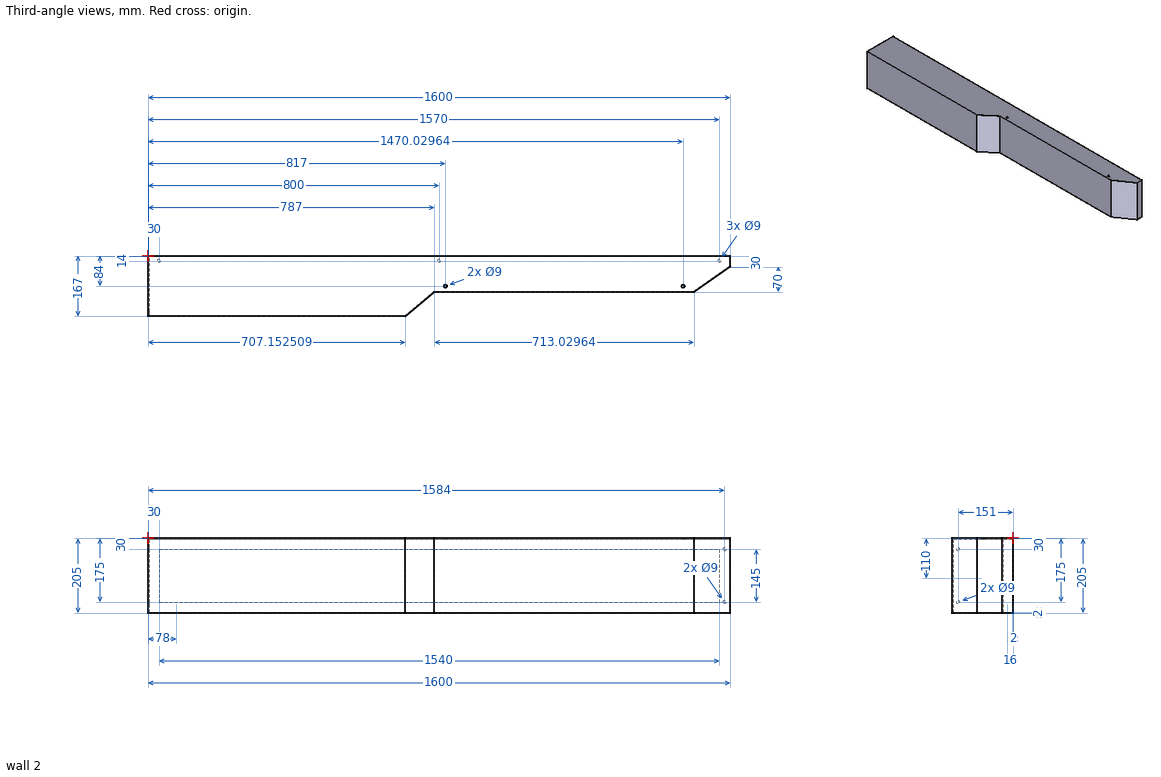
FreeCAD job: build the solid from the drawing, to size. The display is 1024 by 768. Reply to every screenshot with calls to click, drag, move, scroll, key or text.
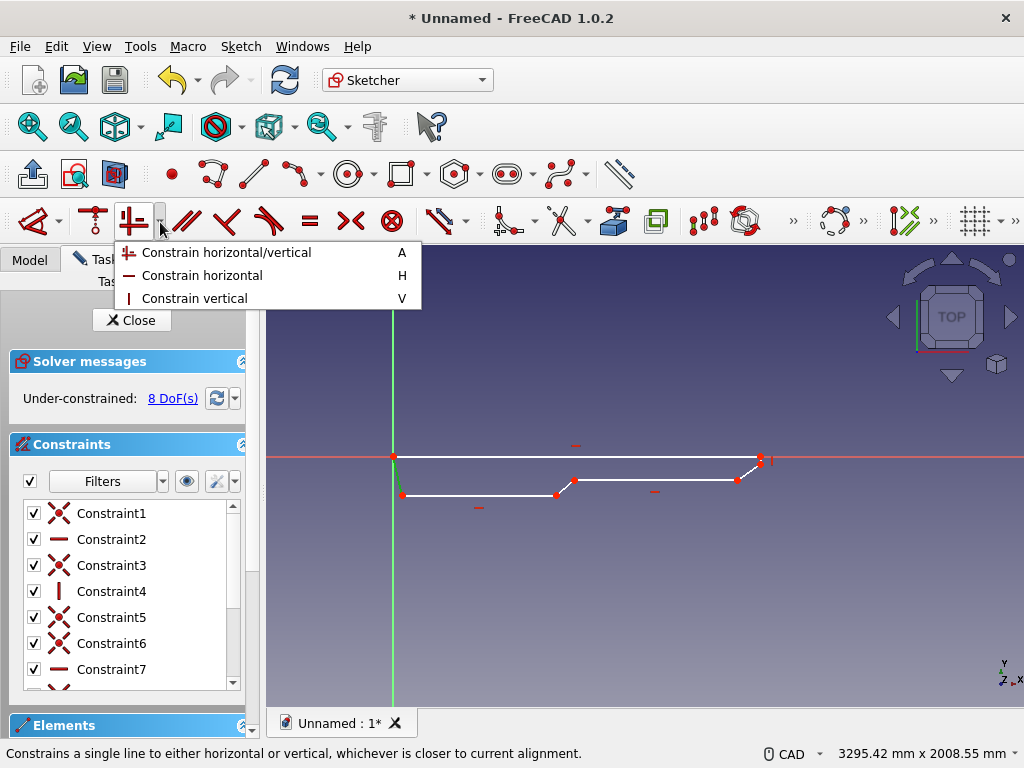
click(268, 298)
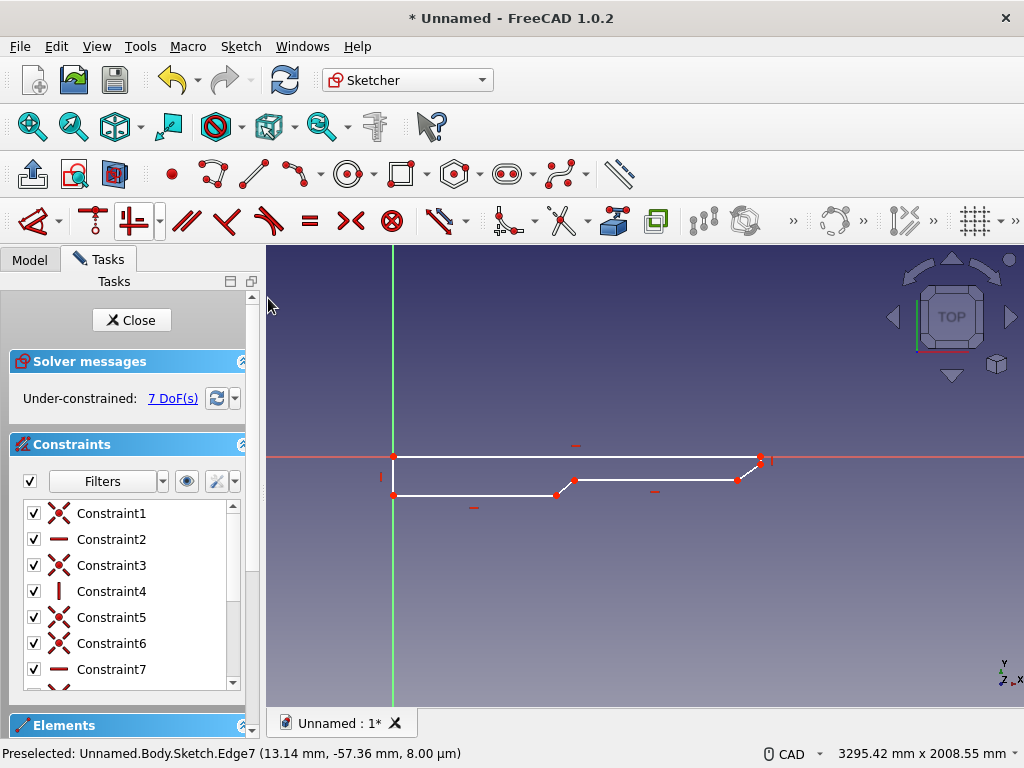
key(d)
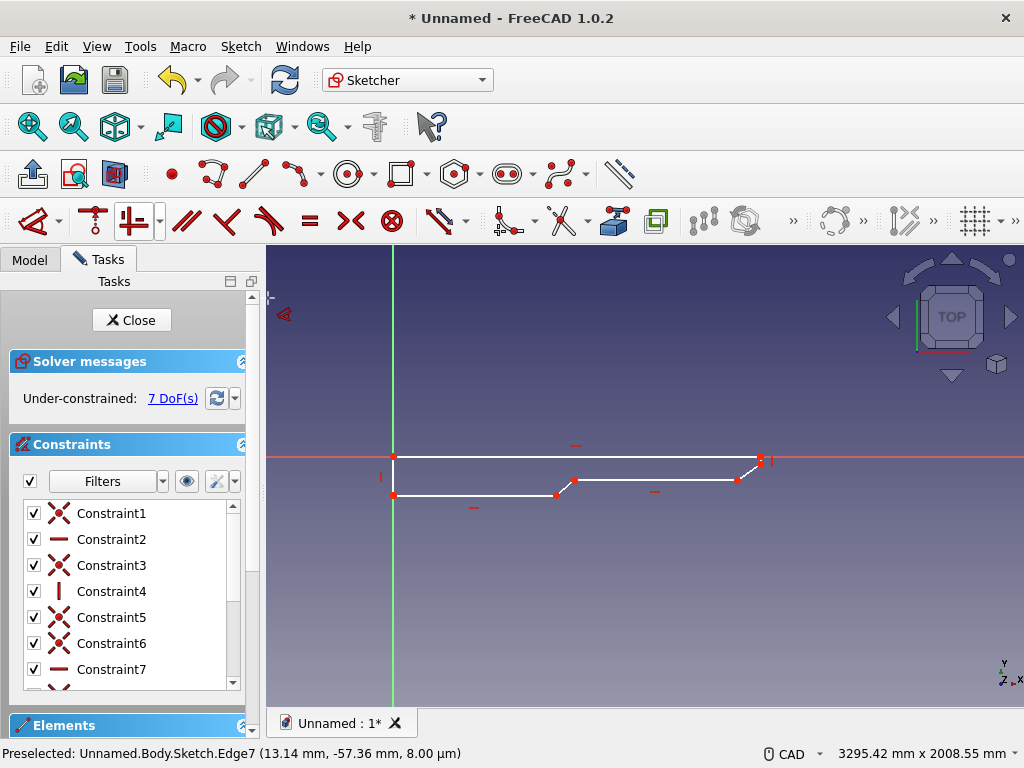
scroll(761, 460, up, 9)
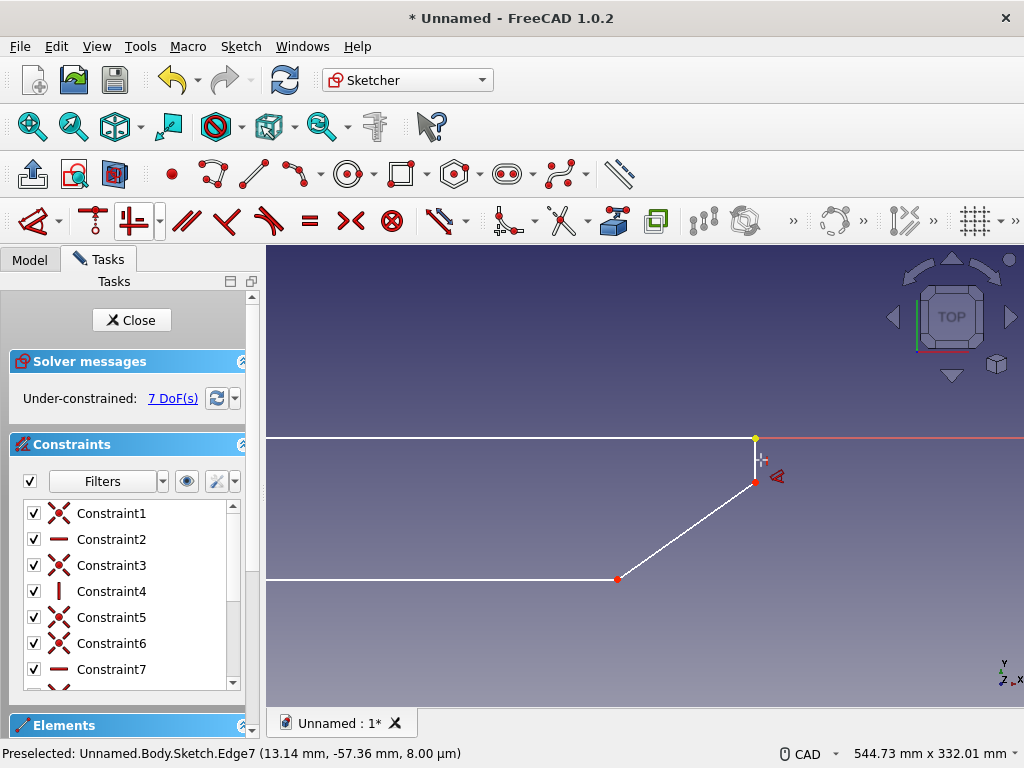
click(755, 460)
click(789, 460)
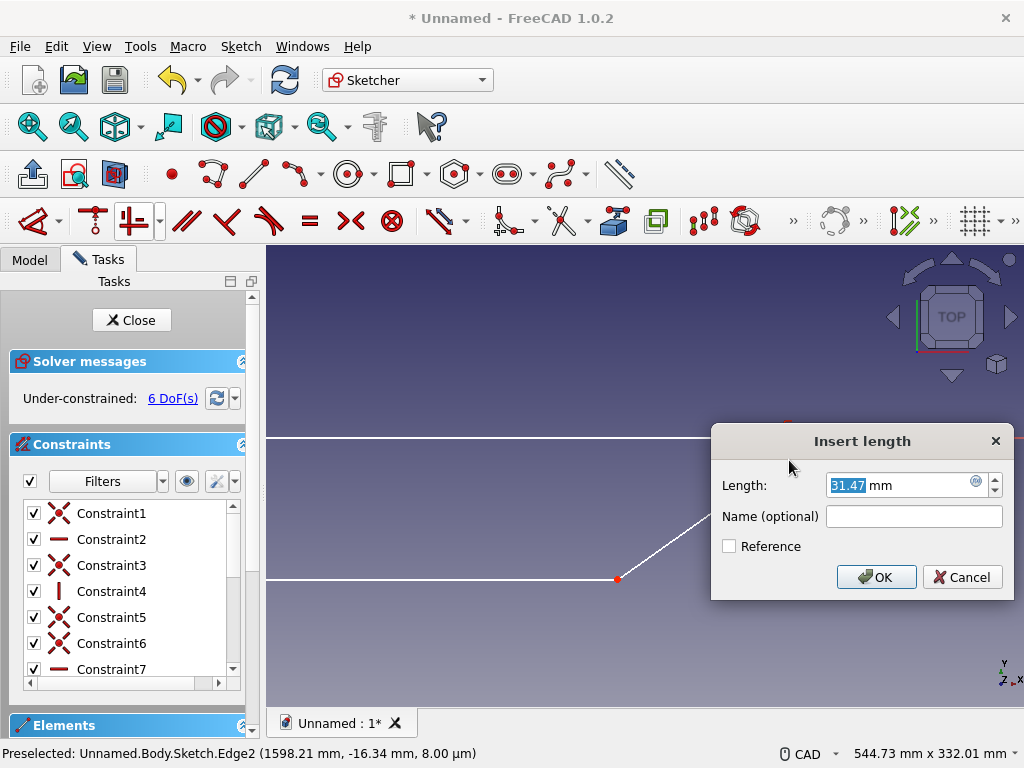
text(30)
key(Return)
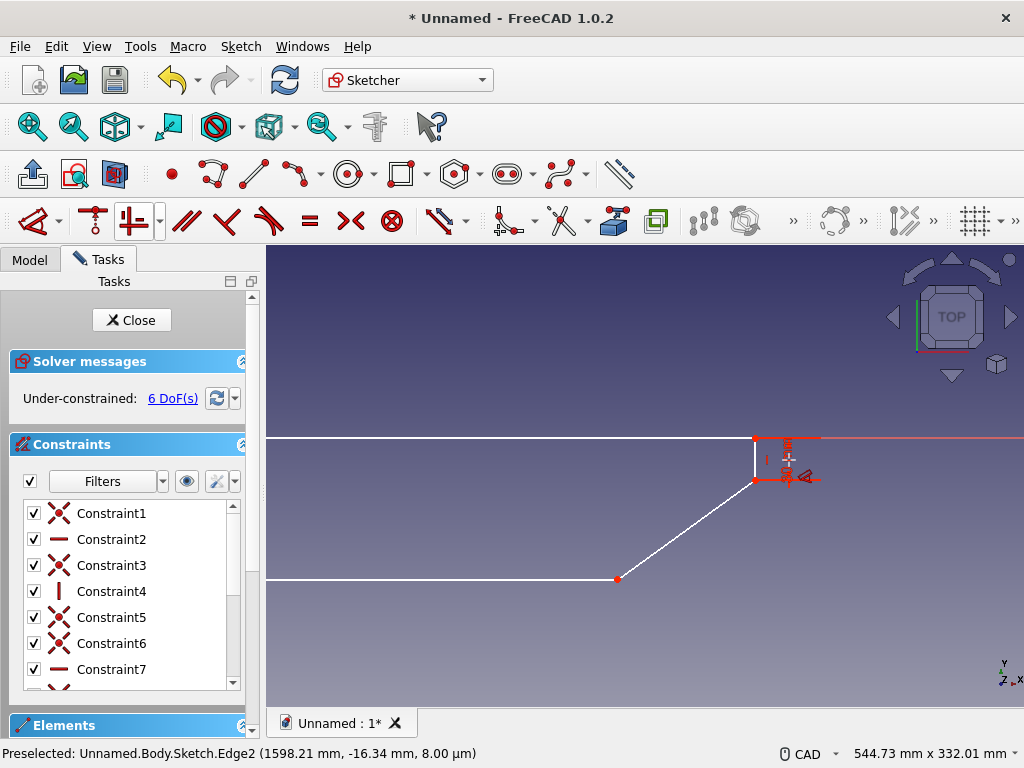
scroll(761, 460, down, 9)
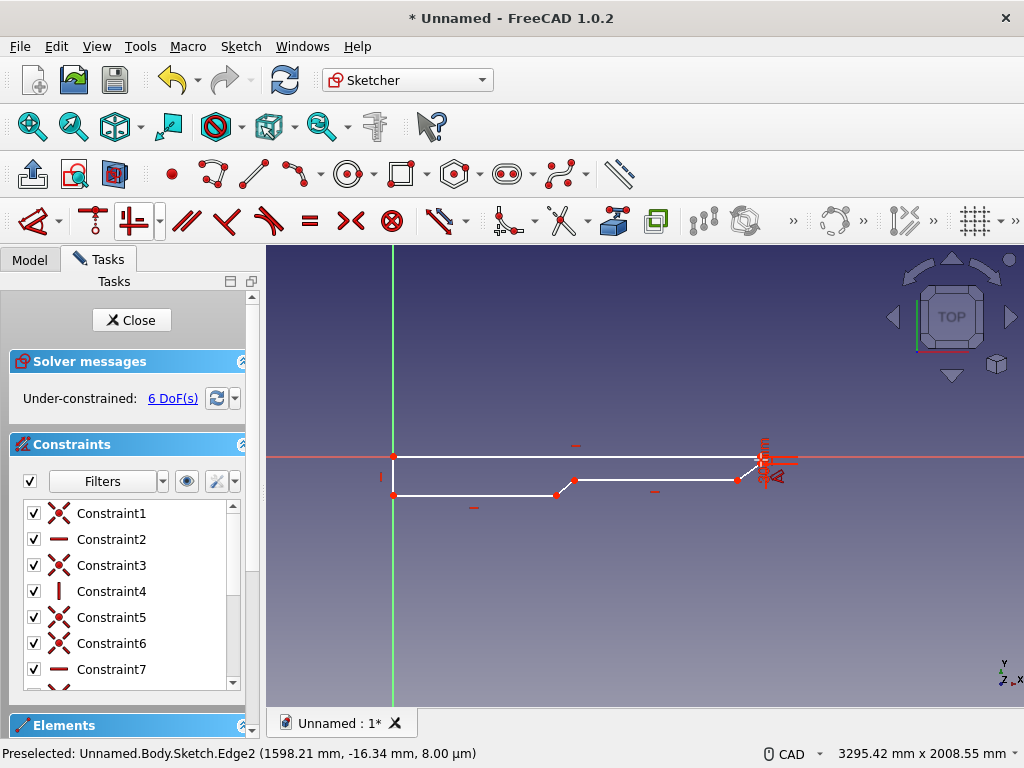
click(393, 484)
click(359, 476)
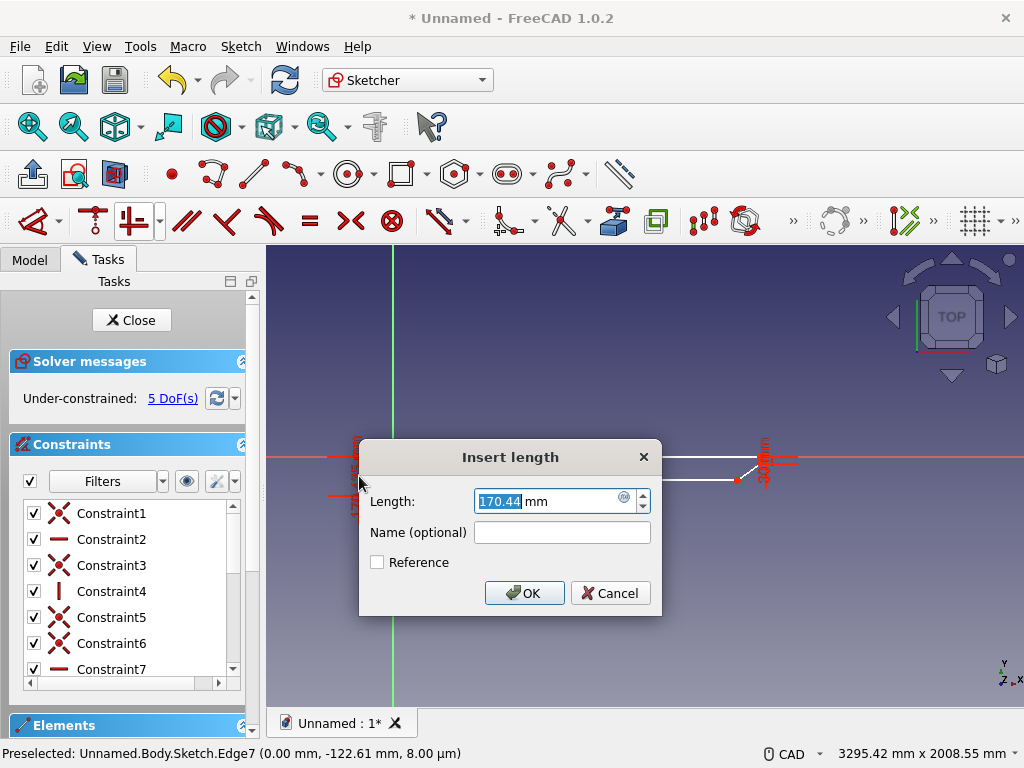
text(167)
key(Return)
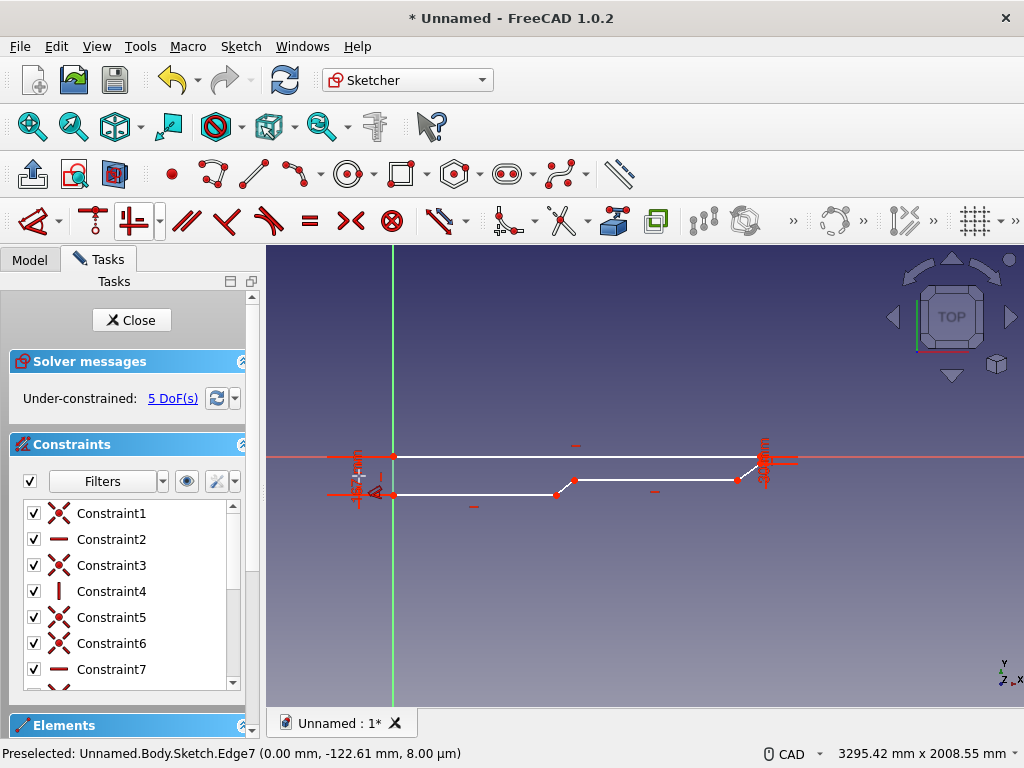
scroll(752, 470, up, 5)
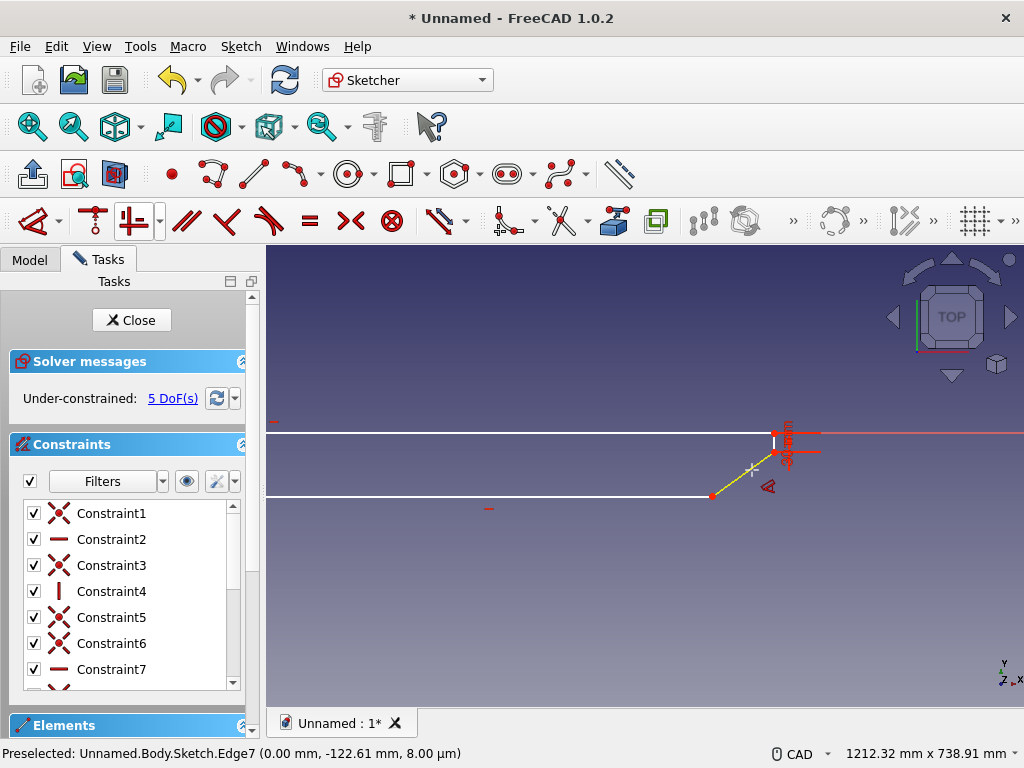
click(750, 470)
click(808, 474)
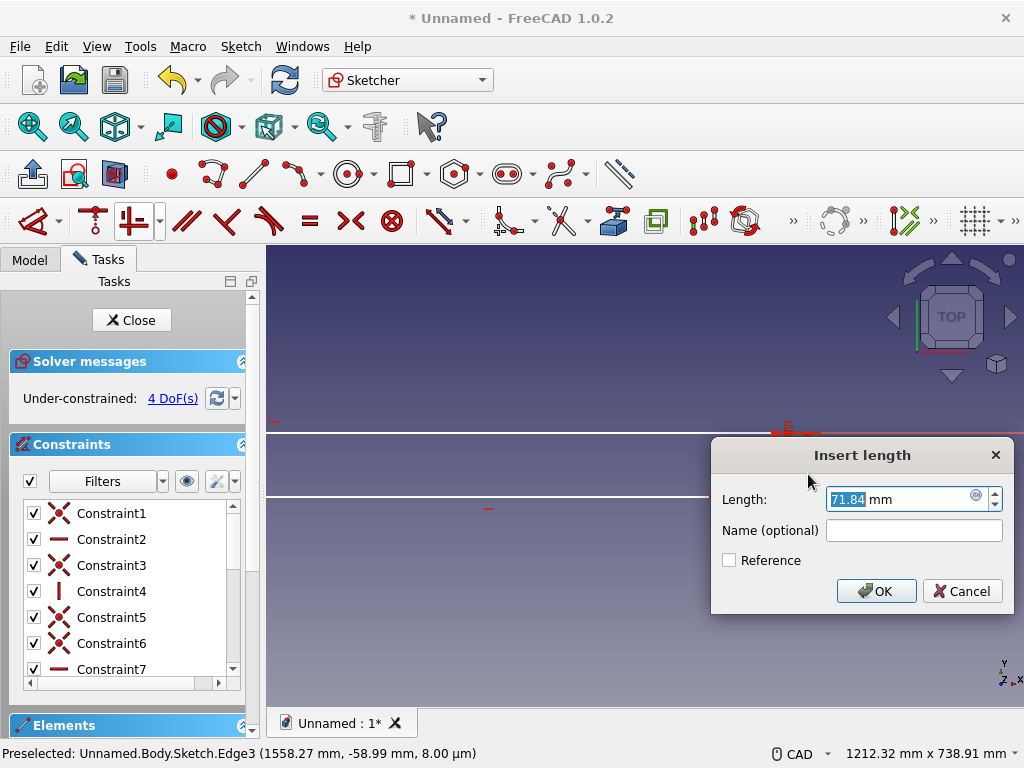
text(70)
key(Return)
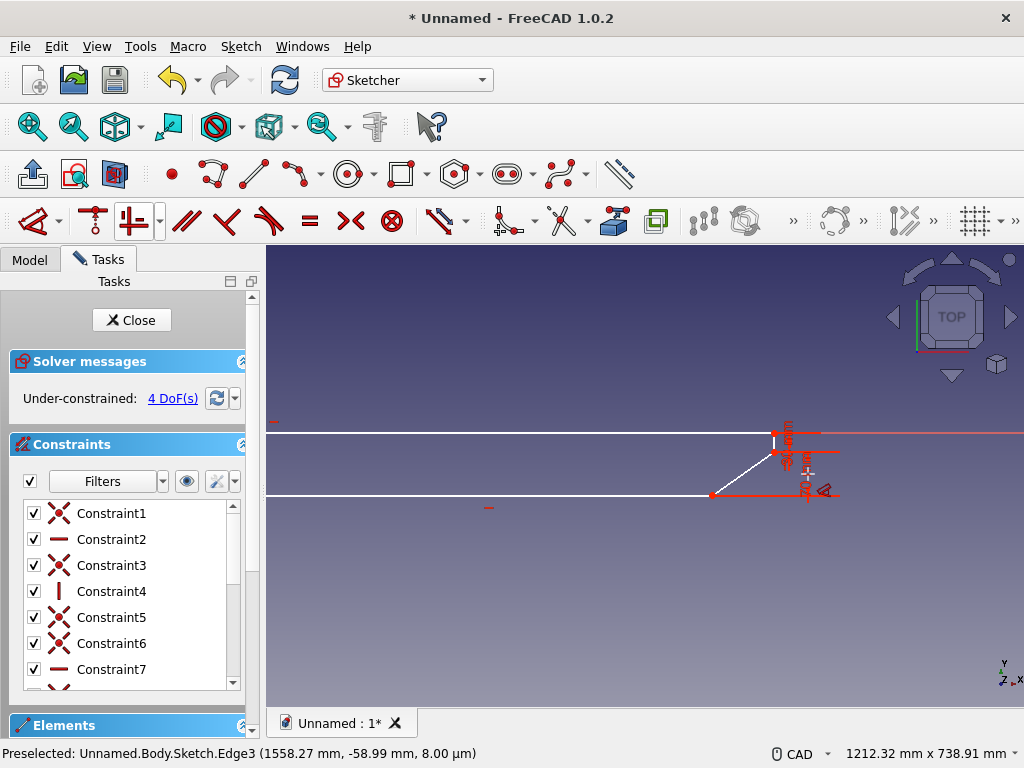
click(475, 433)
click(534, 399)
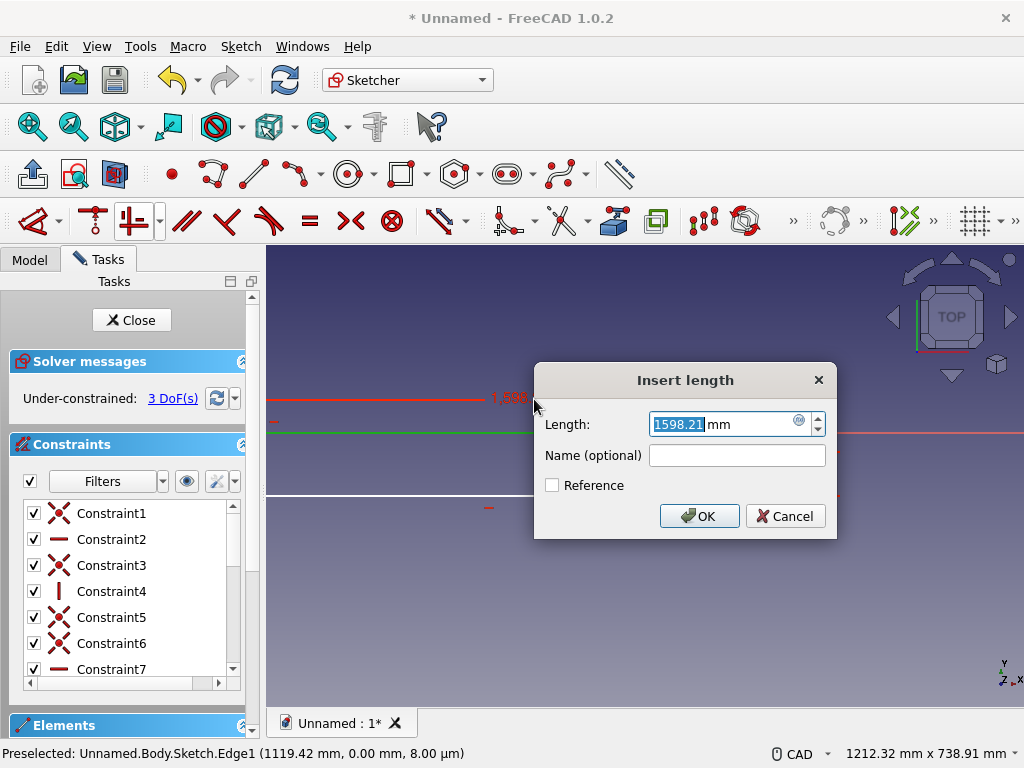
text(1600)
key(Return)